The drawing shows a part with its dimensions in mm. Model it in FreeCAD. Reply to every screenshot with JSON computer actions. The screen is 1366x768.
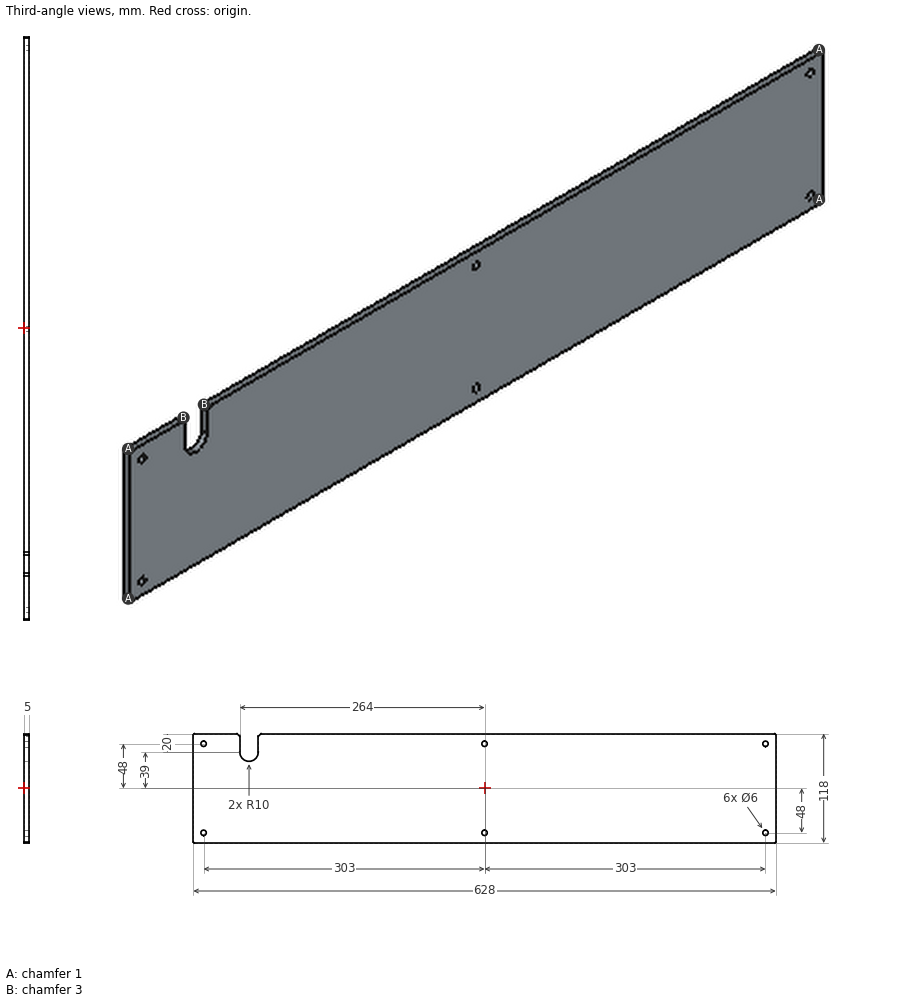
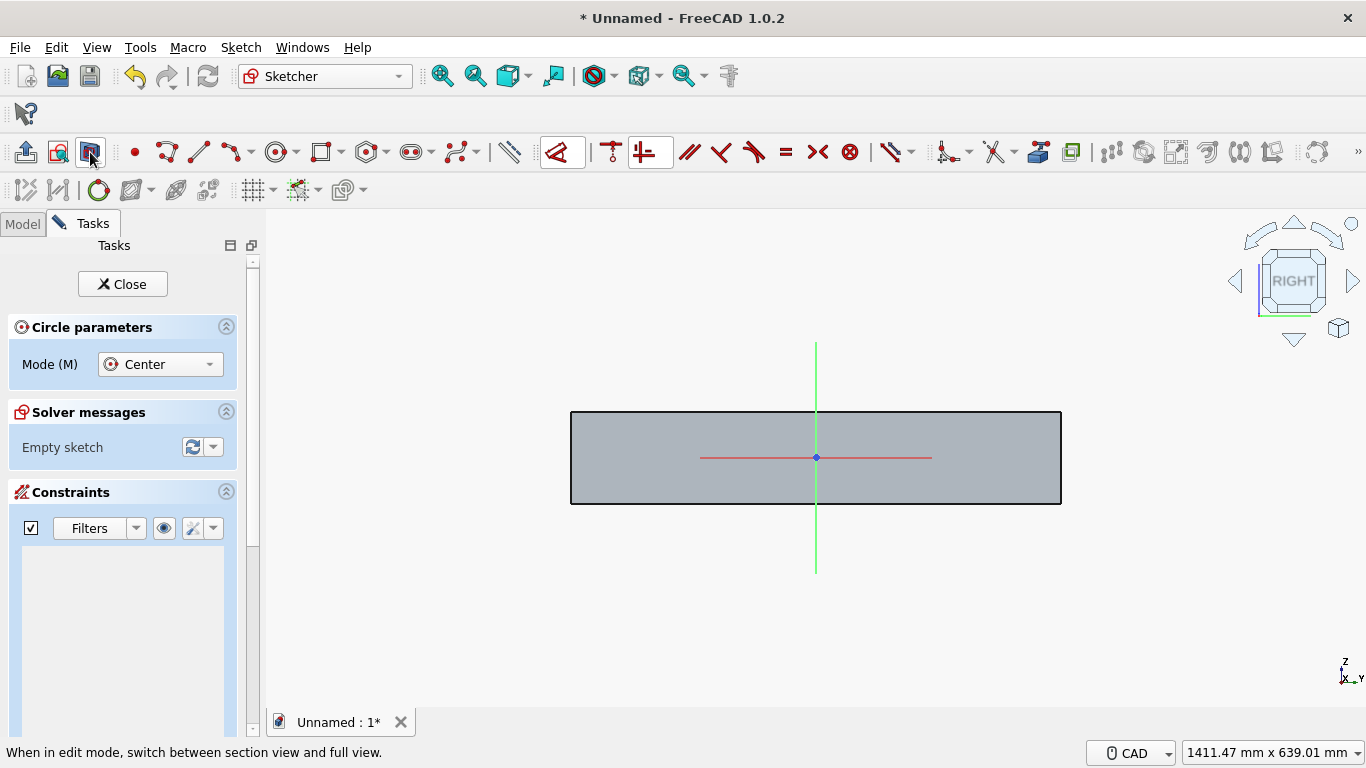
{"action": "scroll", "coordinate": [1052, 495], "scroll_direction": "up", "scroll_amount": 12}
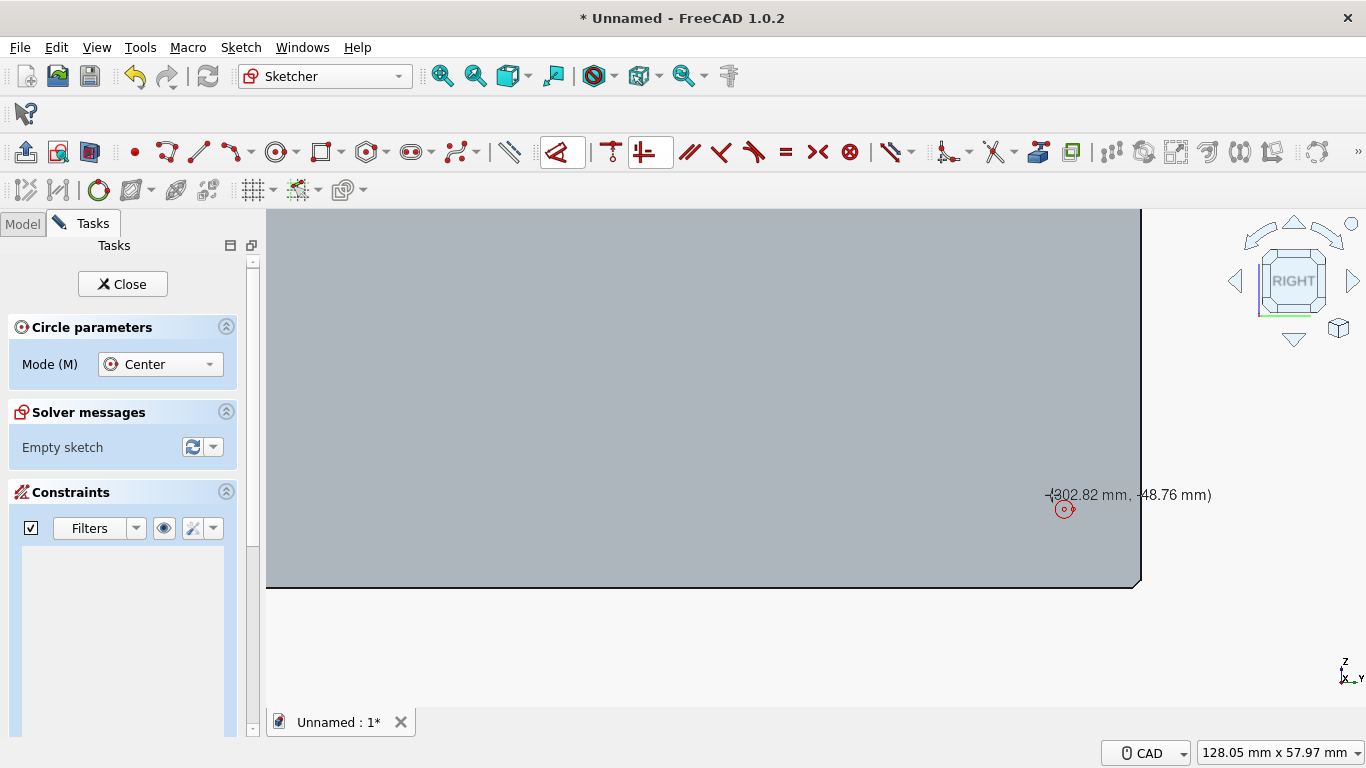
{"action": "scroll", "coordinate": [1035, 505], "scroll_direction": "down", "scroll_amount": 11}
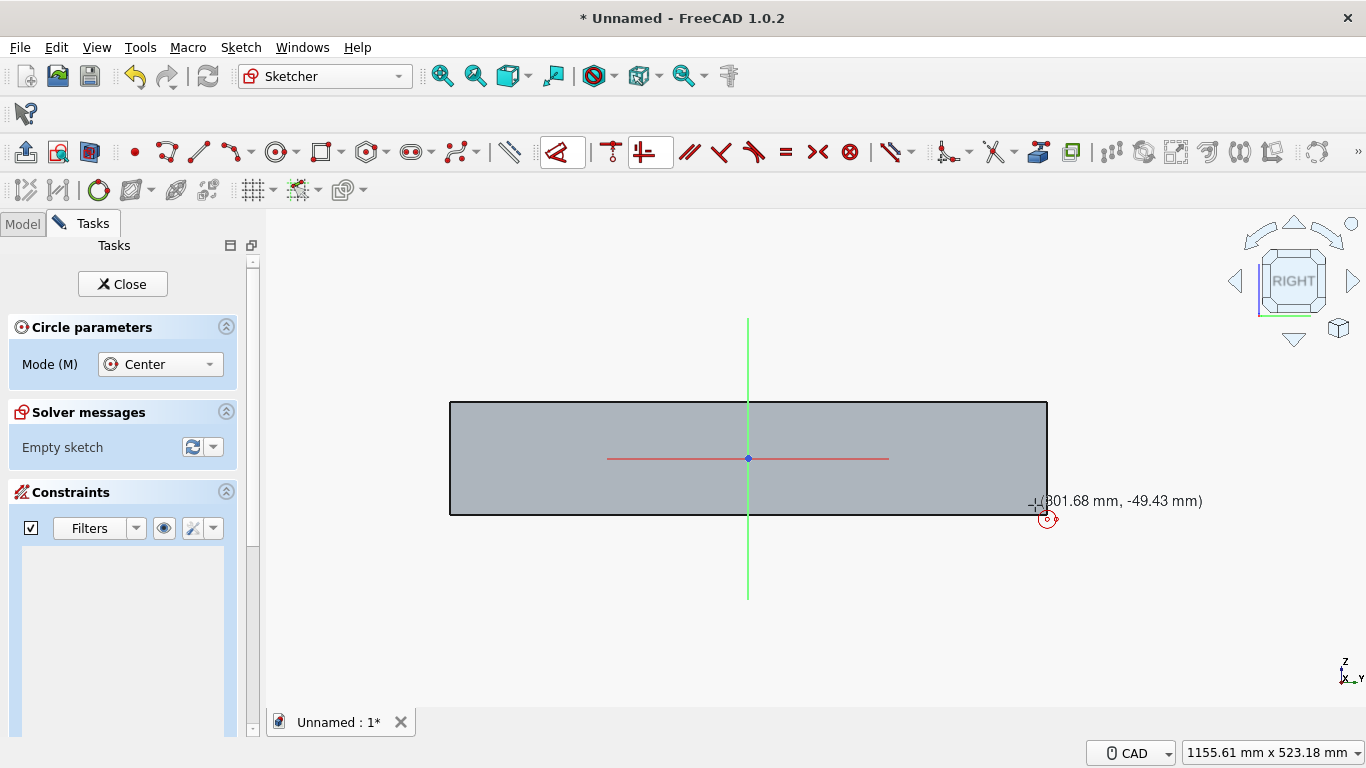
{"action": "left_click", "coordinate": [1037, 504]}
{"action": "mouse_move", "coordinate": [1039, 502]}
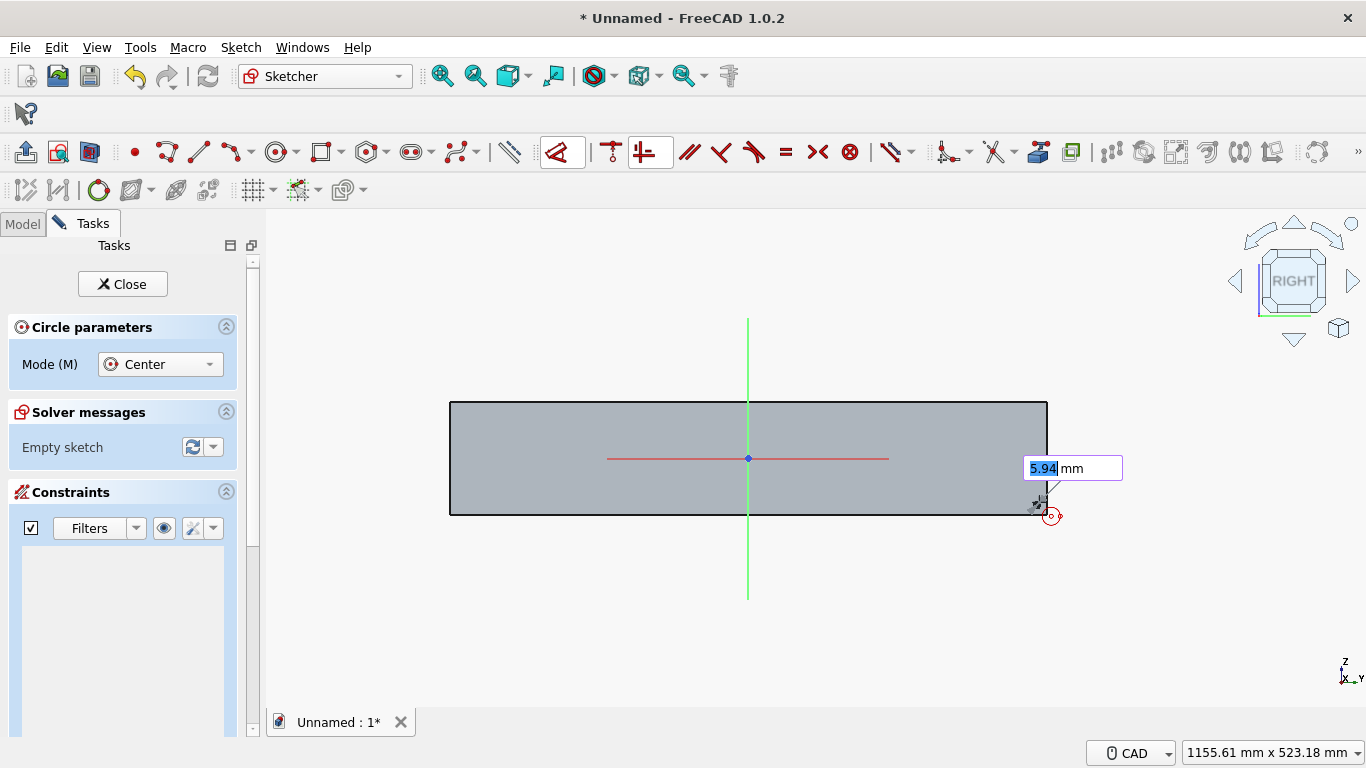
{"action": "type", "text": "6"}
{"action": "key", "text": "Return"}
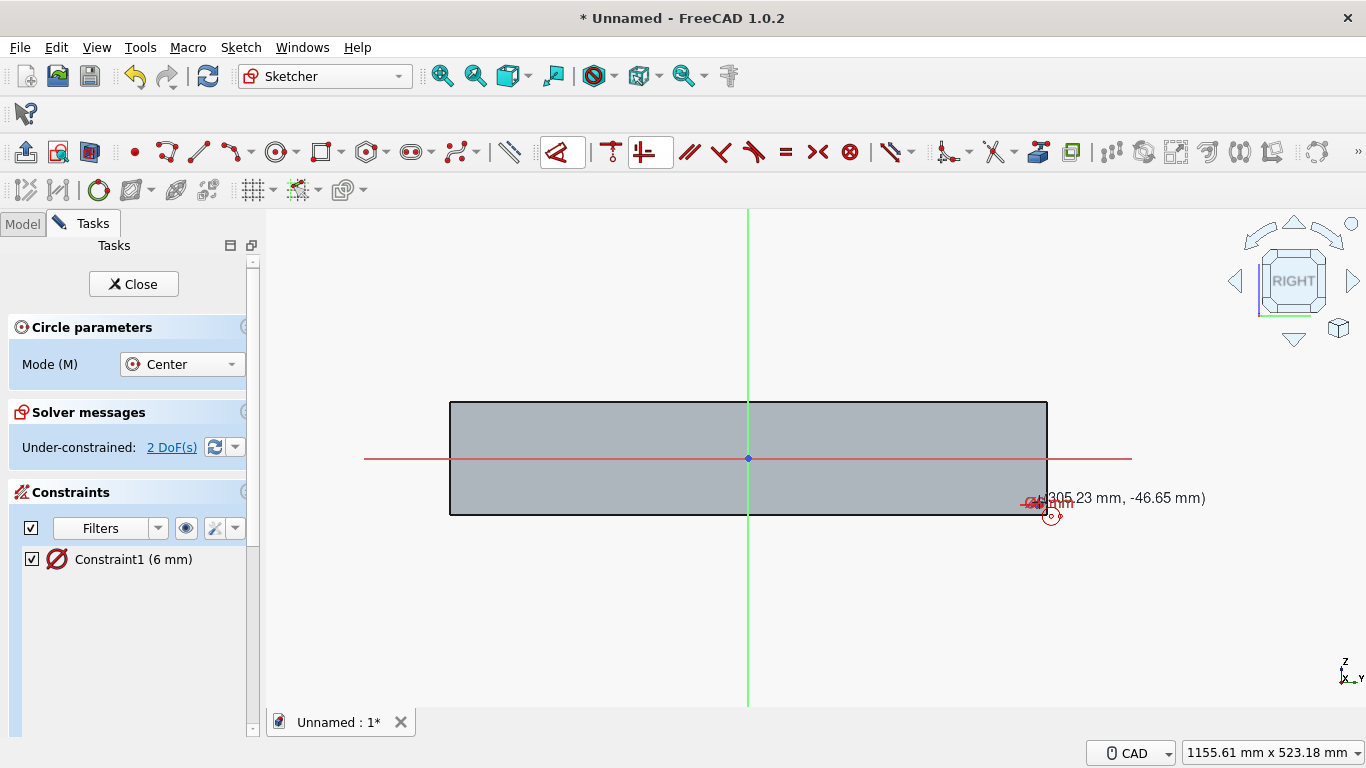
{"action": "scroll", "coordinate": [460, 504], "scroll_direction": "up", "scroll_amount": 11}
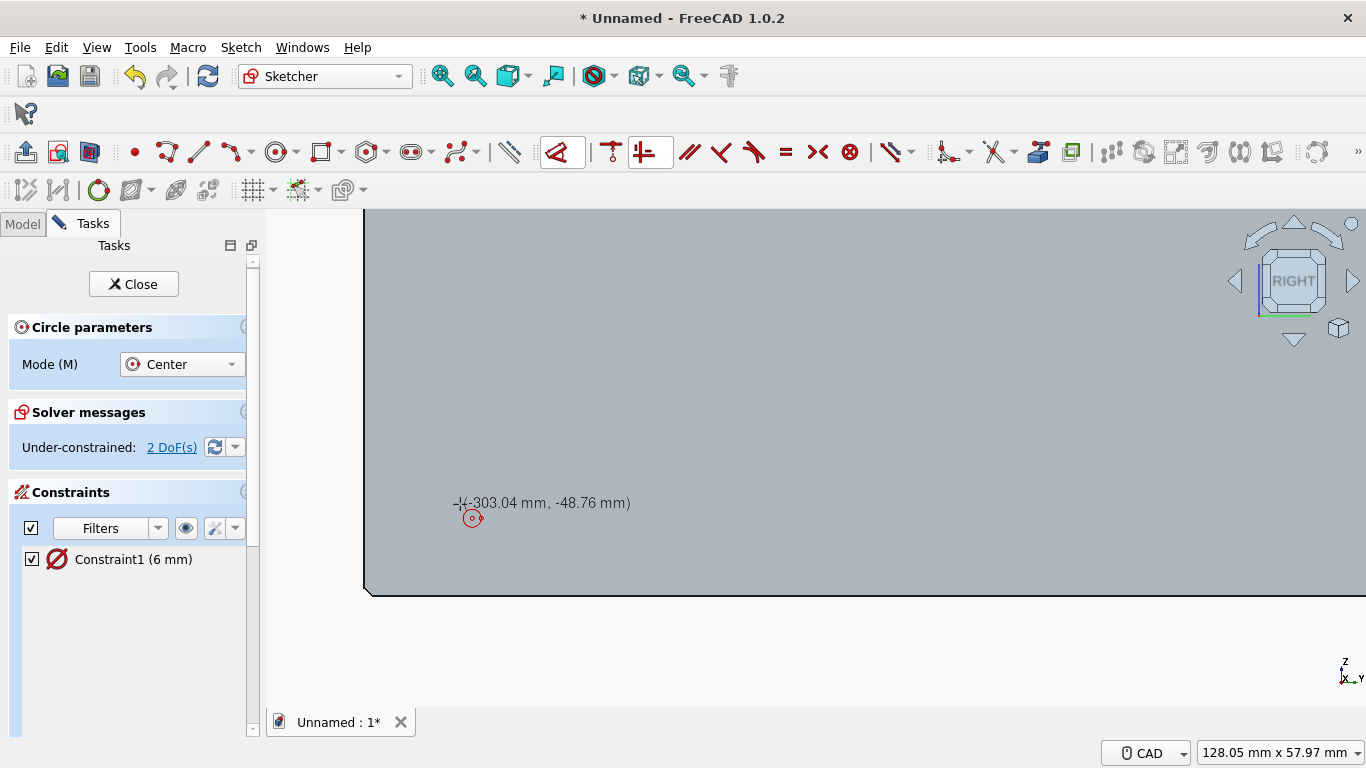
{"action": "scroll", "coordinate": [459, 504], "scroll_direction": "down", "scroll_amount": 11}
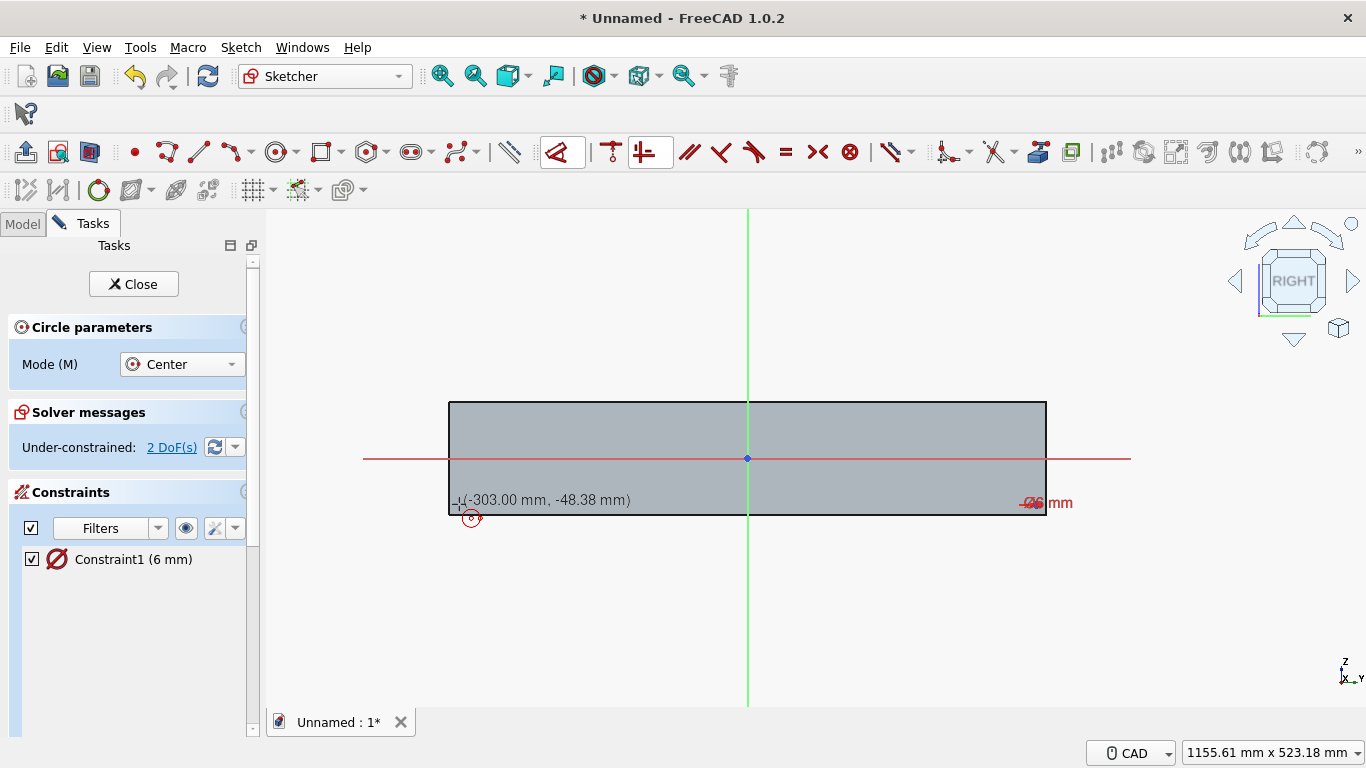
{"action": "left_click", "coordinate": [459, 504]}
{"action": "mouse_move", "coordinate": [461, 502]}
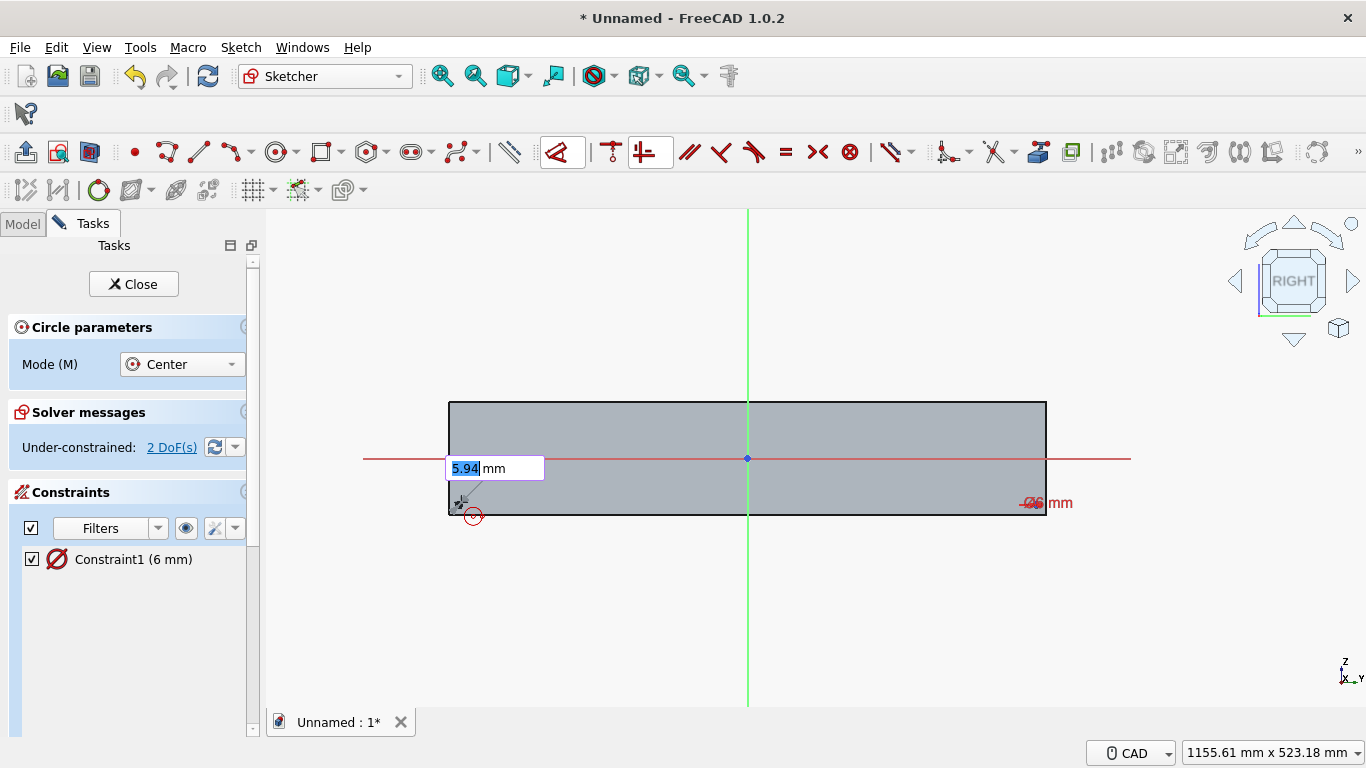
{"action": "type", "text": "6"}
{"action": "key", "text": "Return"}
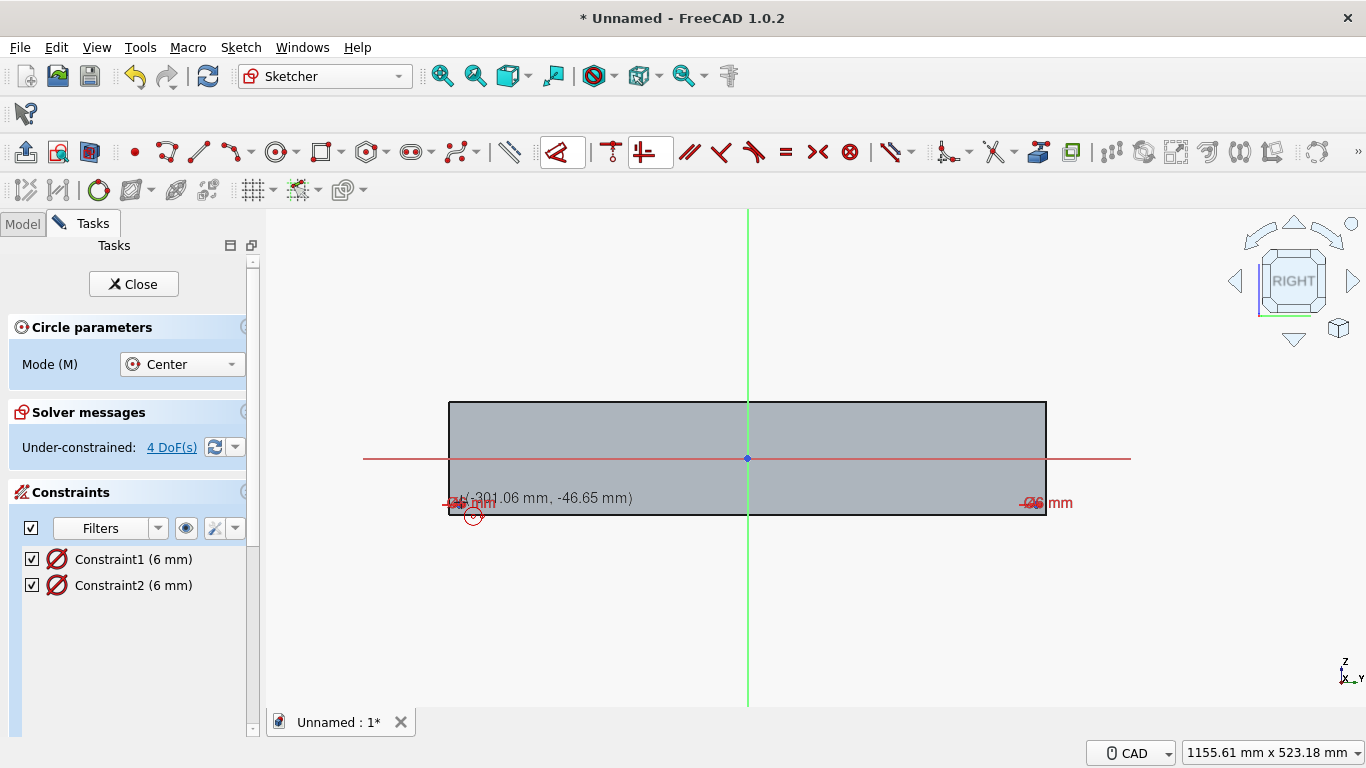
{"action": "scroll", "coordinate": [459, 413], "scroll_direction": "up", "scroll_amount": 11}